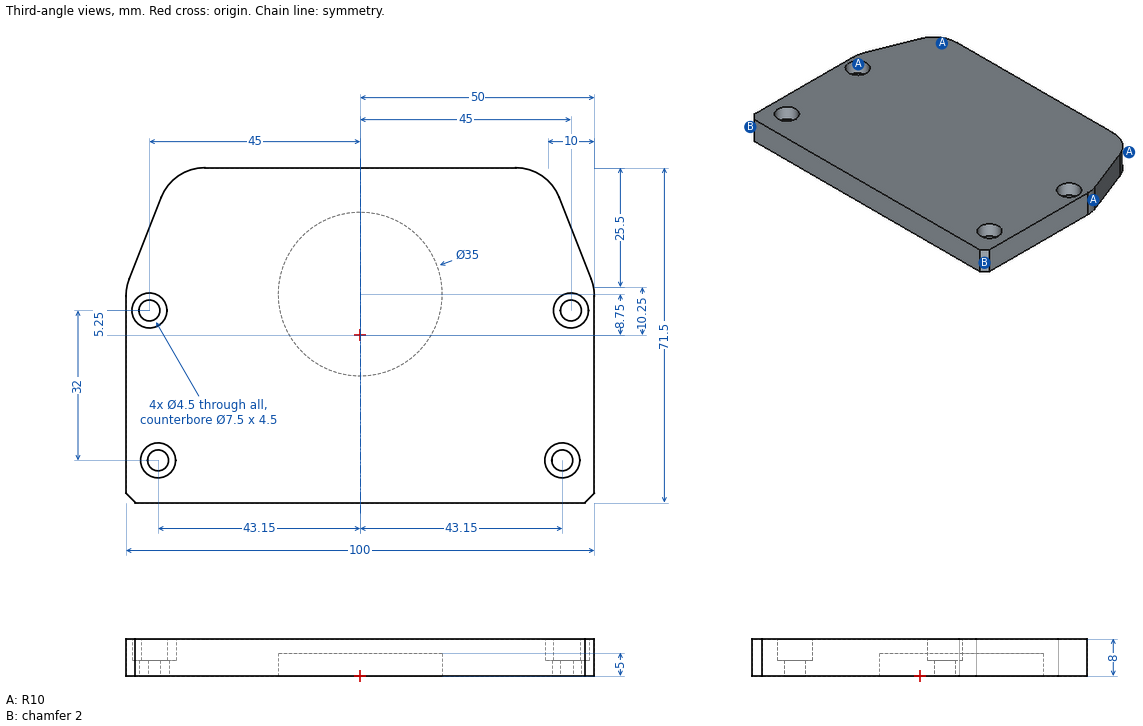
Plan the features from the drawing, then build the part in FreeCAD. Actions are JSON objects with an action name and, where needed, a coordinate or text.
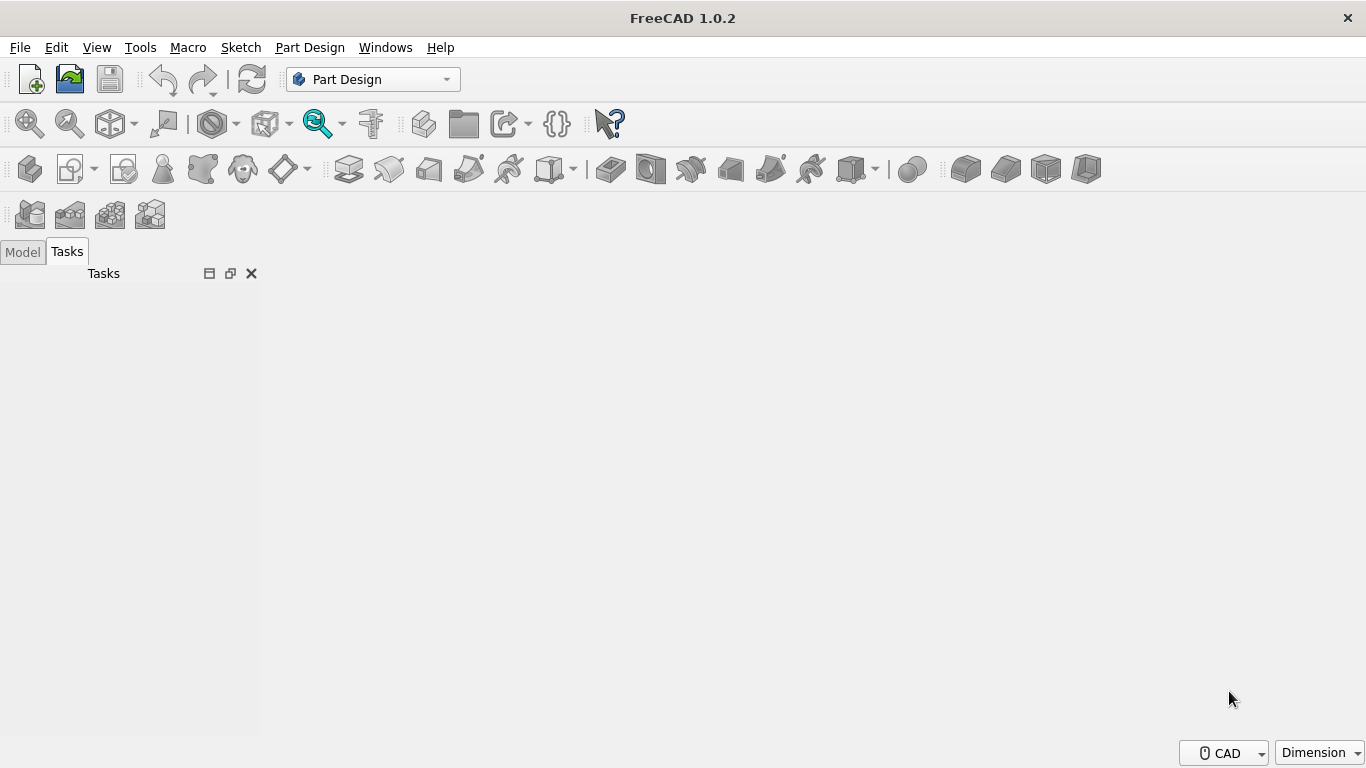
{"action": "left_click", "coordinate": [30, 80]}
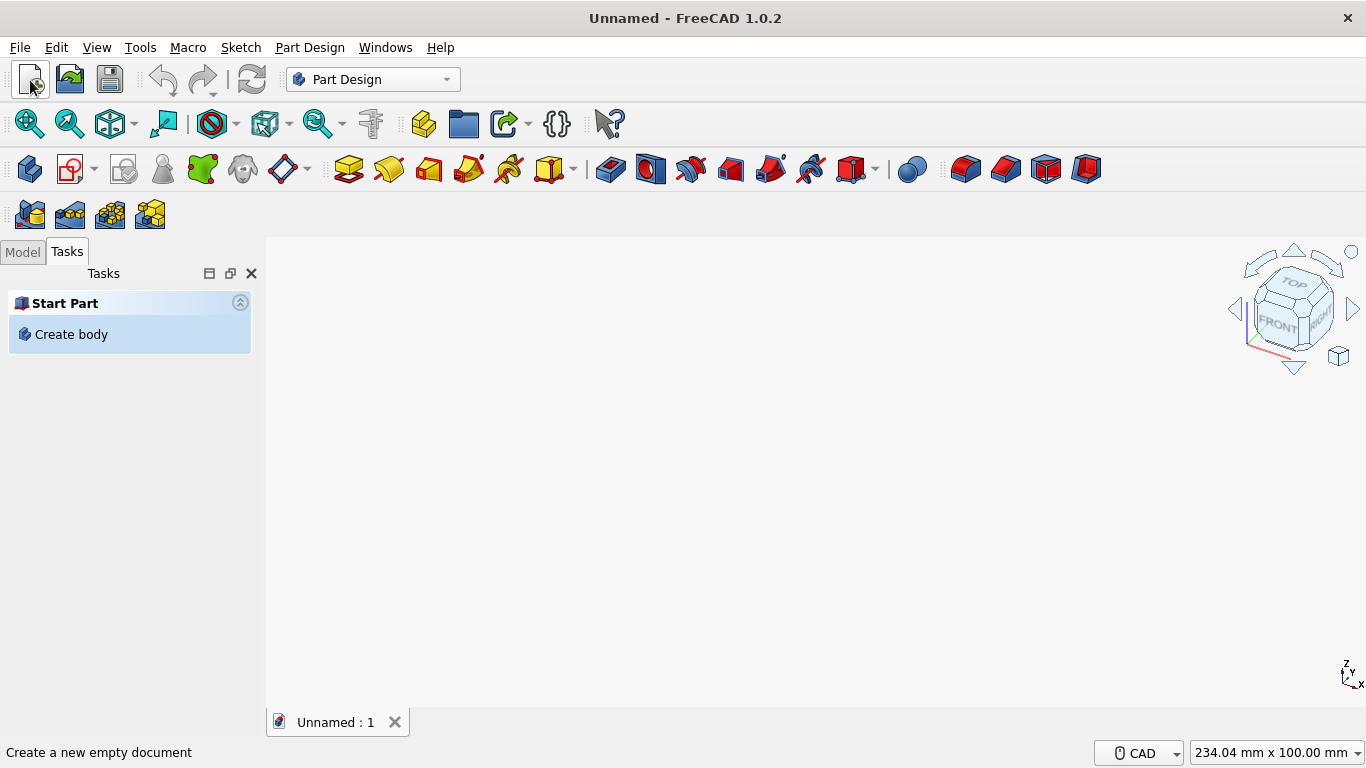
{"action": "left_click", "coordinate": [70, 170]}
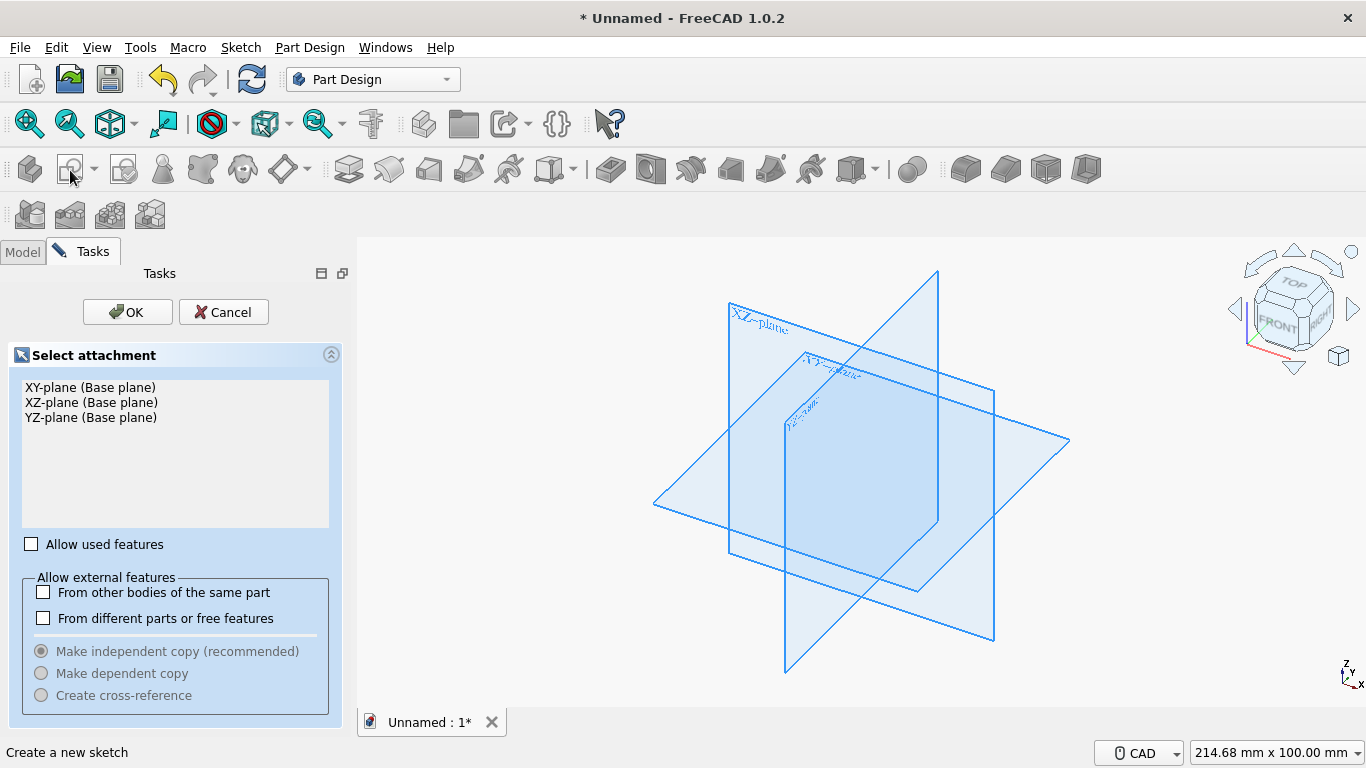
{"action": "left_click", "coordinate": [82, 388]}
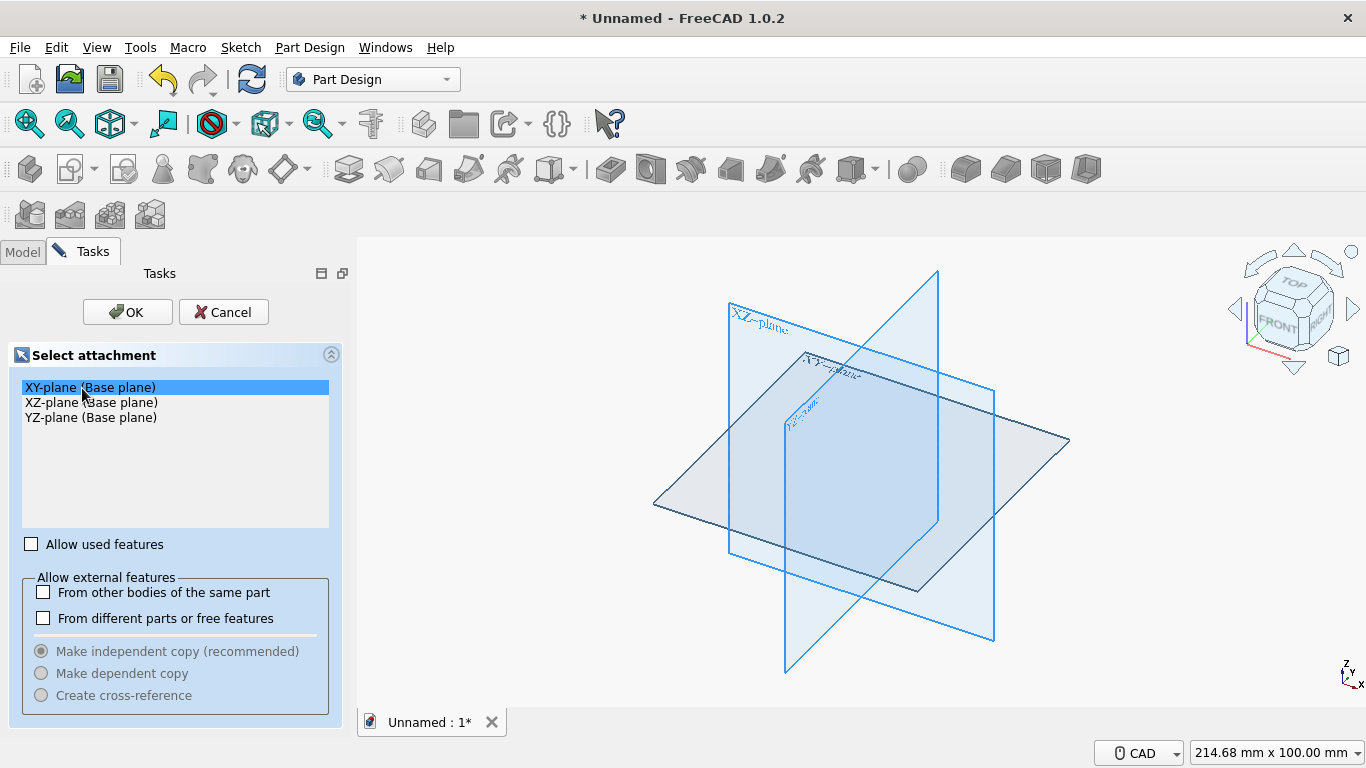
{"action": "left_click", "coordinate": [128, 312]}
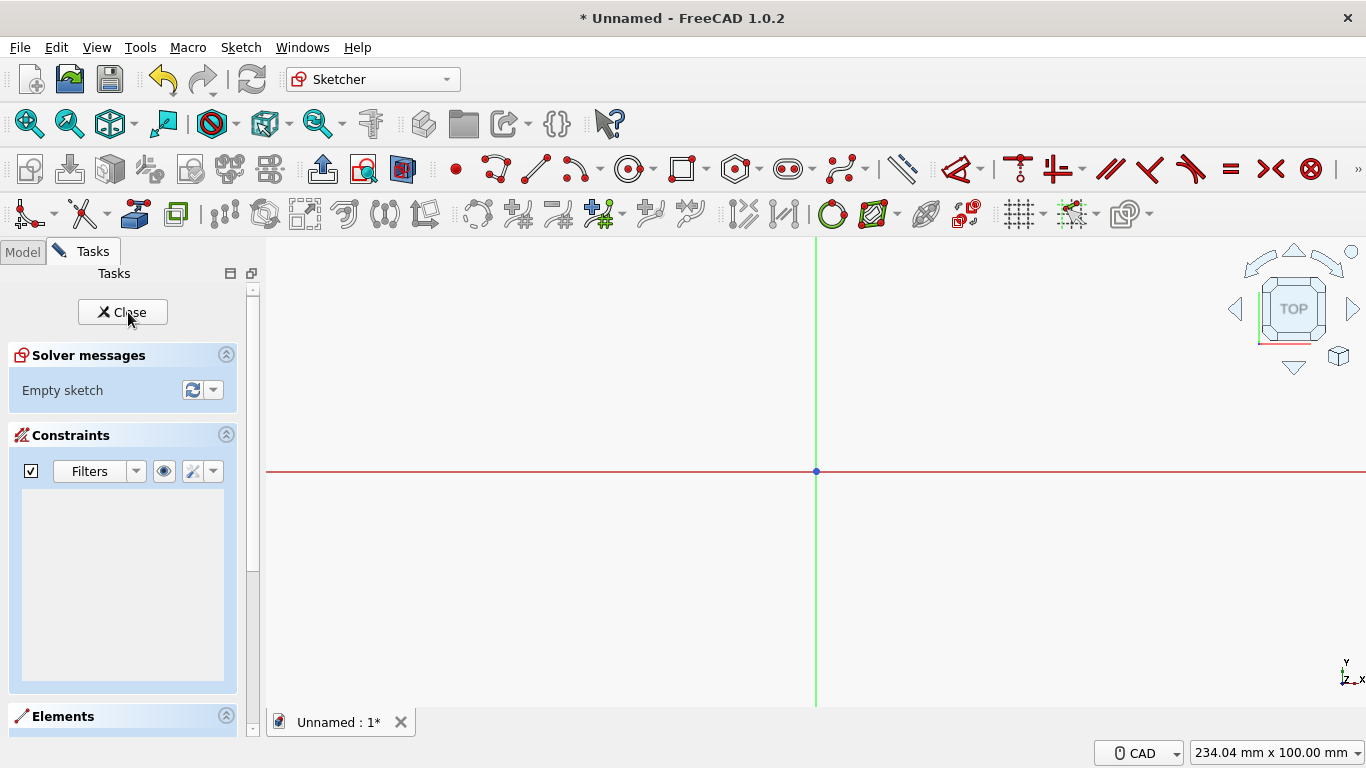
{"action": "left_click", "coordinate": [708, 170]}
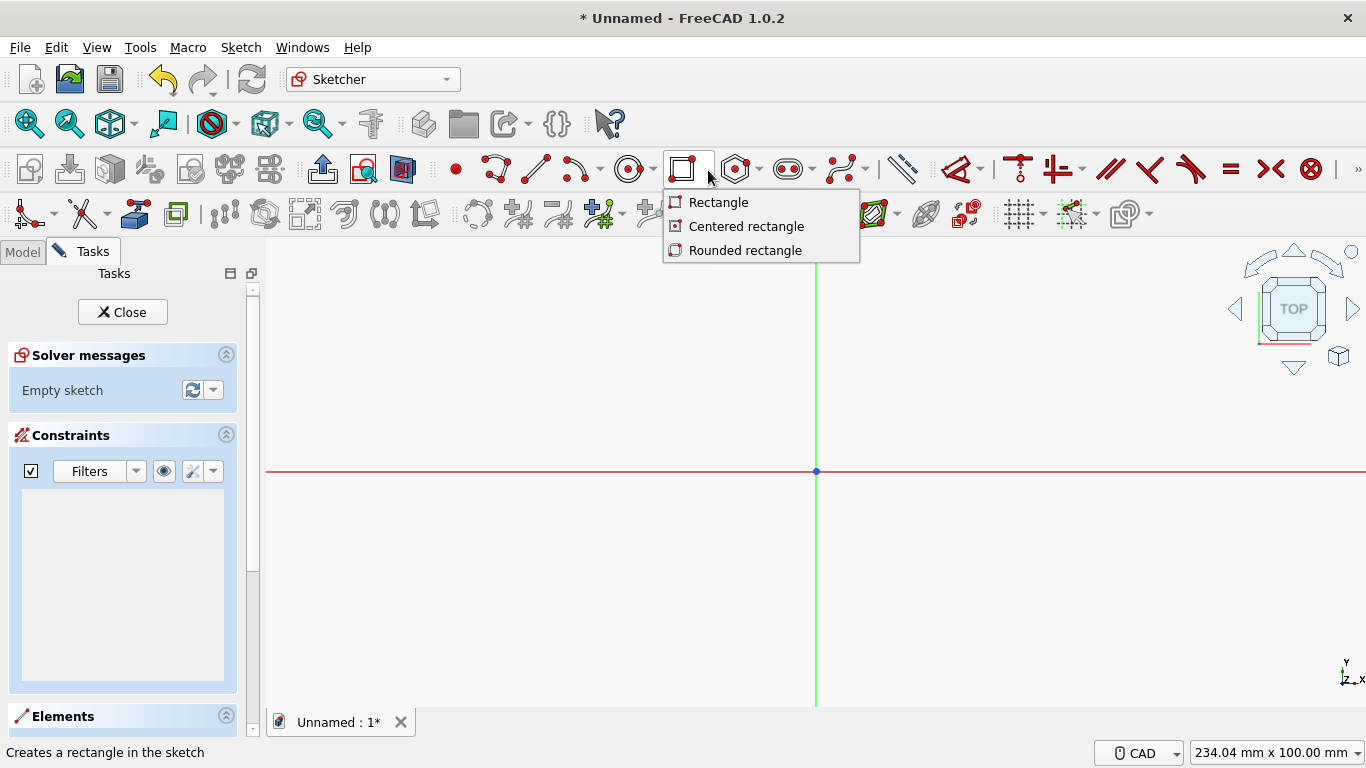
{"action": "left_click", "coordinate": [762, 226]}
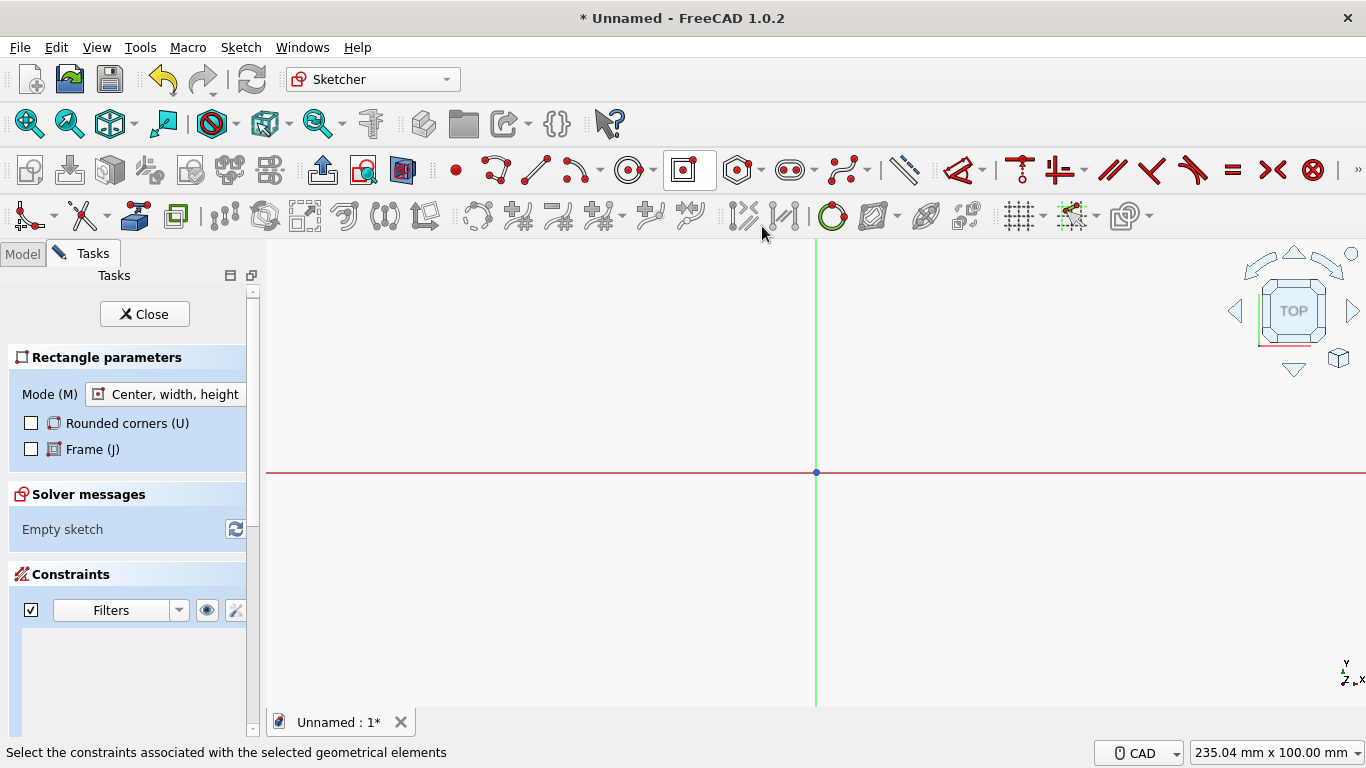
{"action": "left_click", "coordinate": [816, 473]}
{"action": "left_click", "coordinate": [1050, 306]}
{"action": "key", "text": "Escape"}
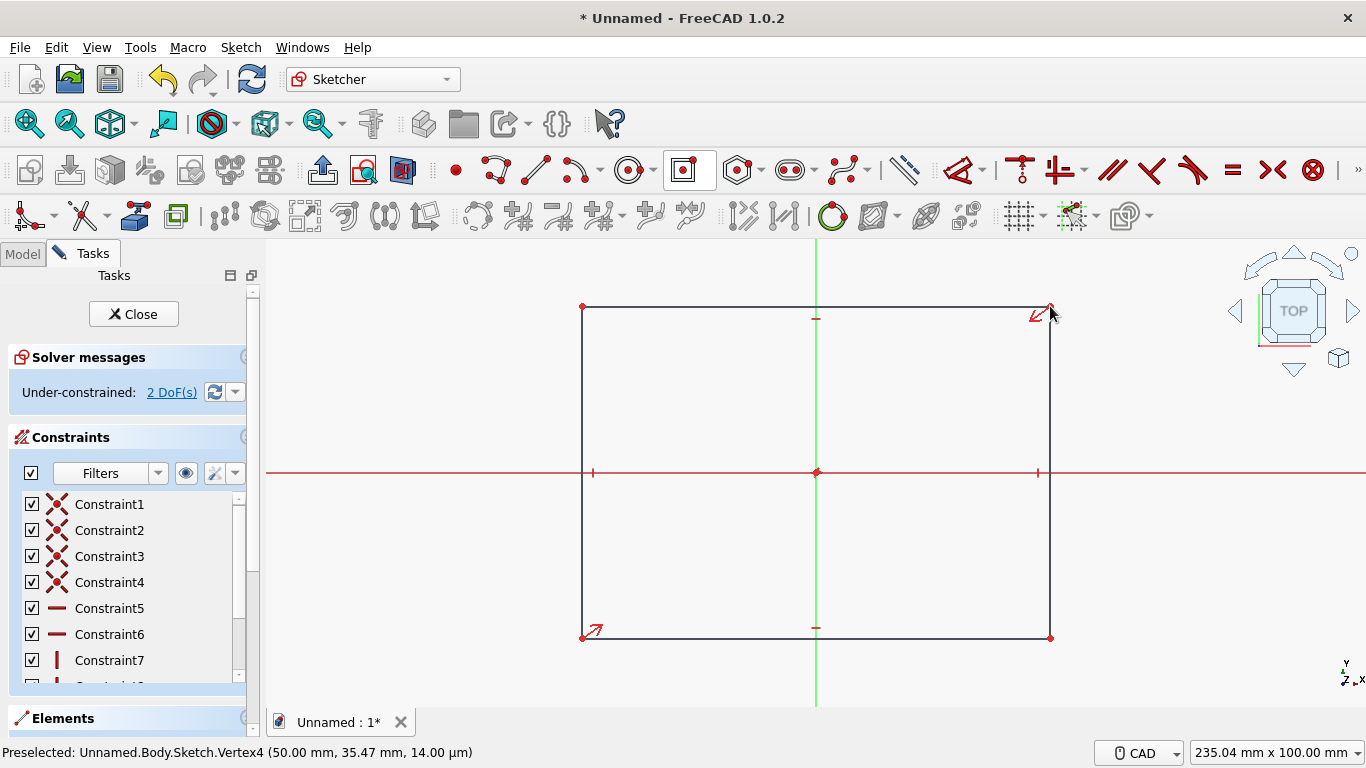
{"action": "left_click", "coordinate": [958, 170]}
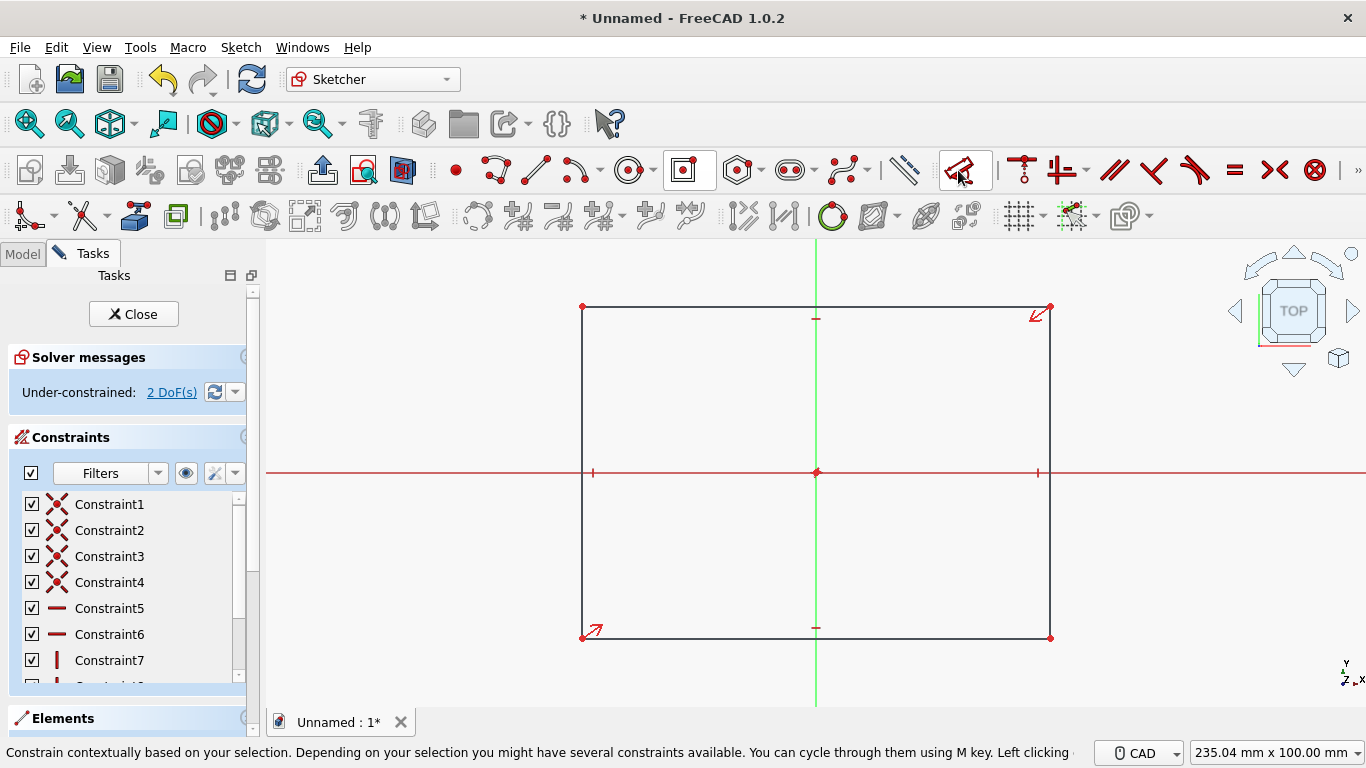
{"action": "left_click", "coordinate": [722, 639]}
{"action": "left_click", "coordinate": [708, 673]}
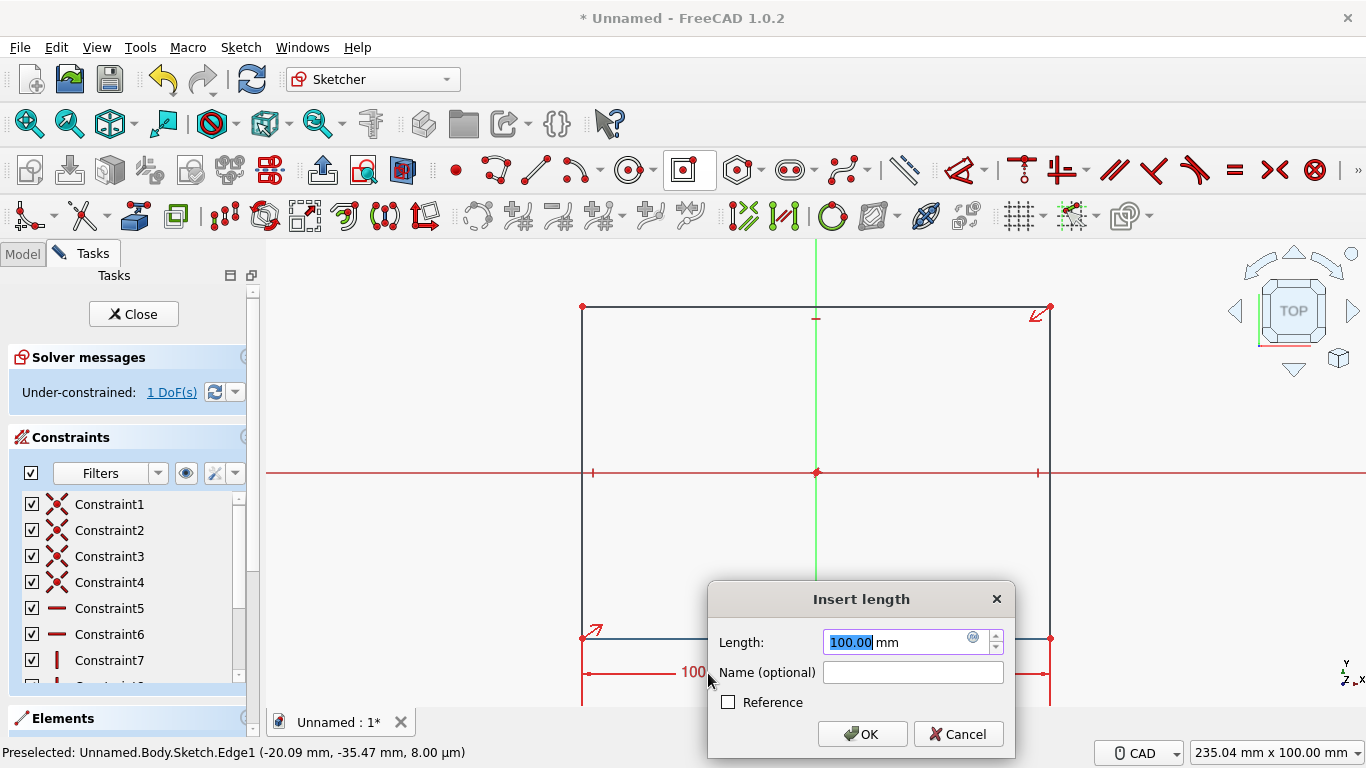
{"action": "type", "text": "100"}
{"action": "key", "text": "Return"}